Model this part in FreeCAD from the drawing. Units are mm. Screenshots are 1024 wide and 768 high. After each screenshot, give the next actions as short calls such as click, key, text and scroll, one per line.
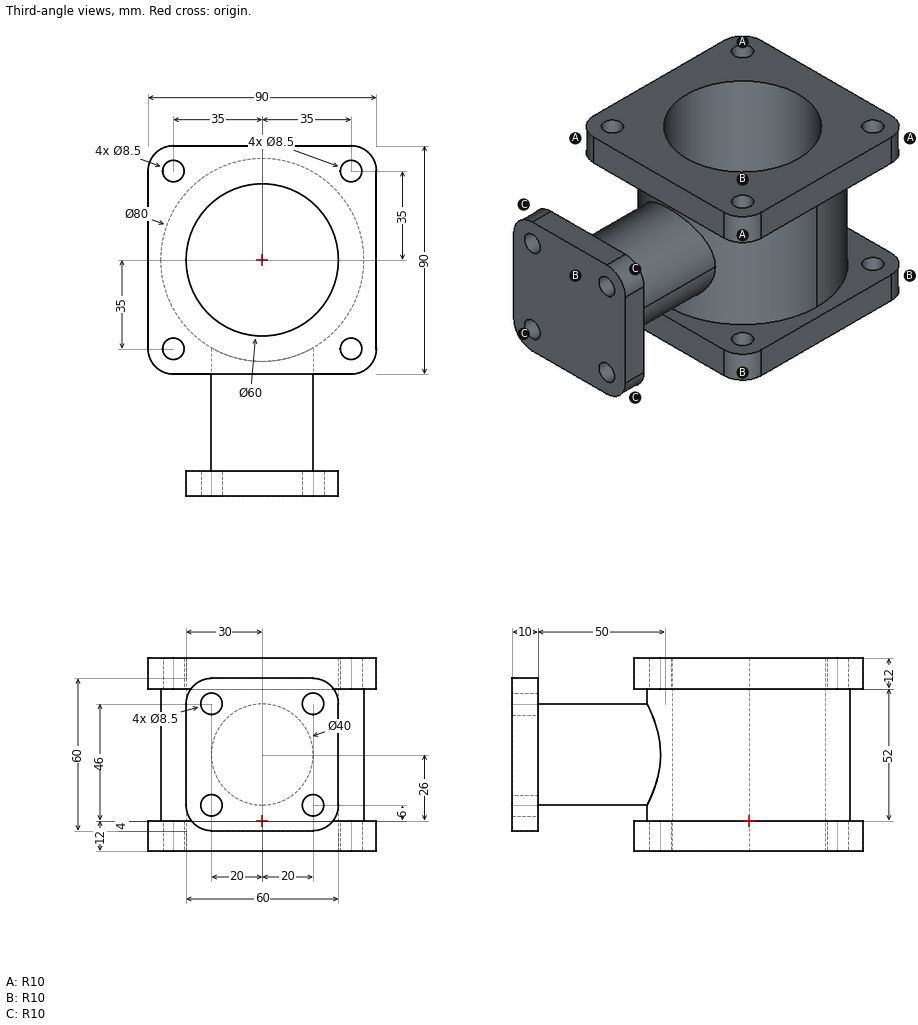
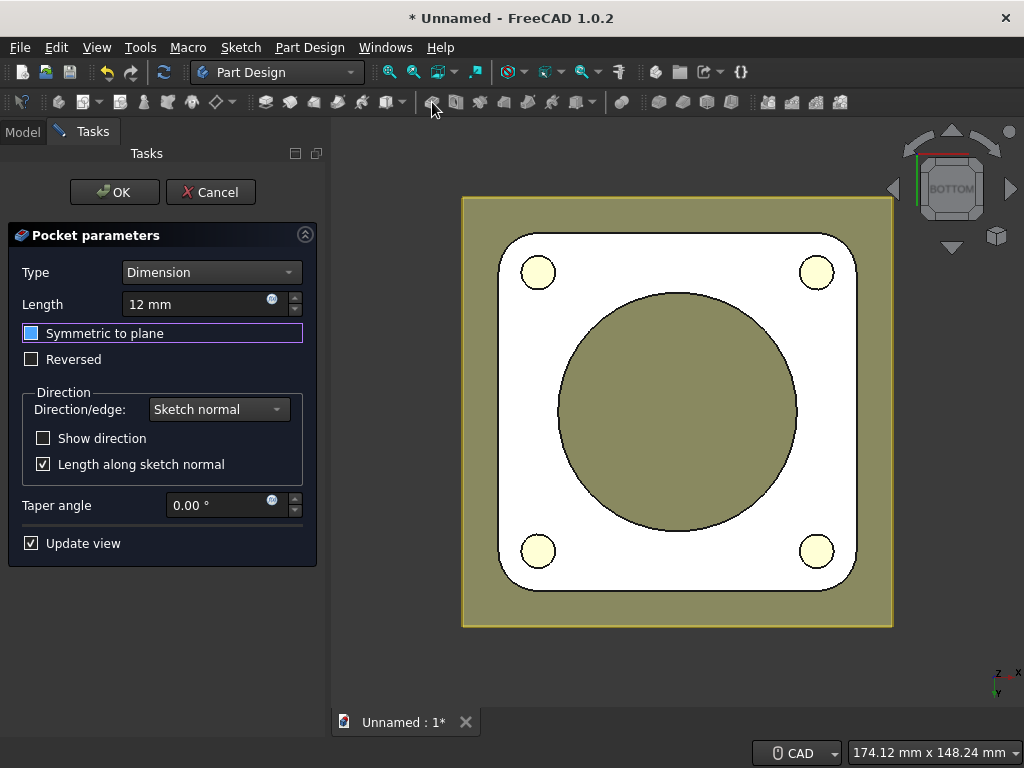
click(30, 359)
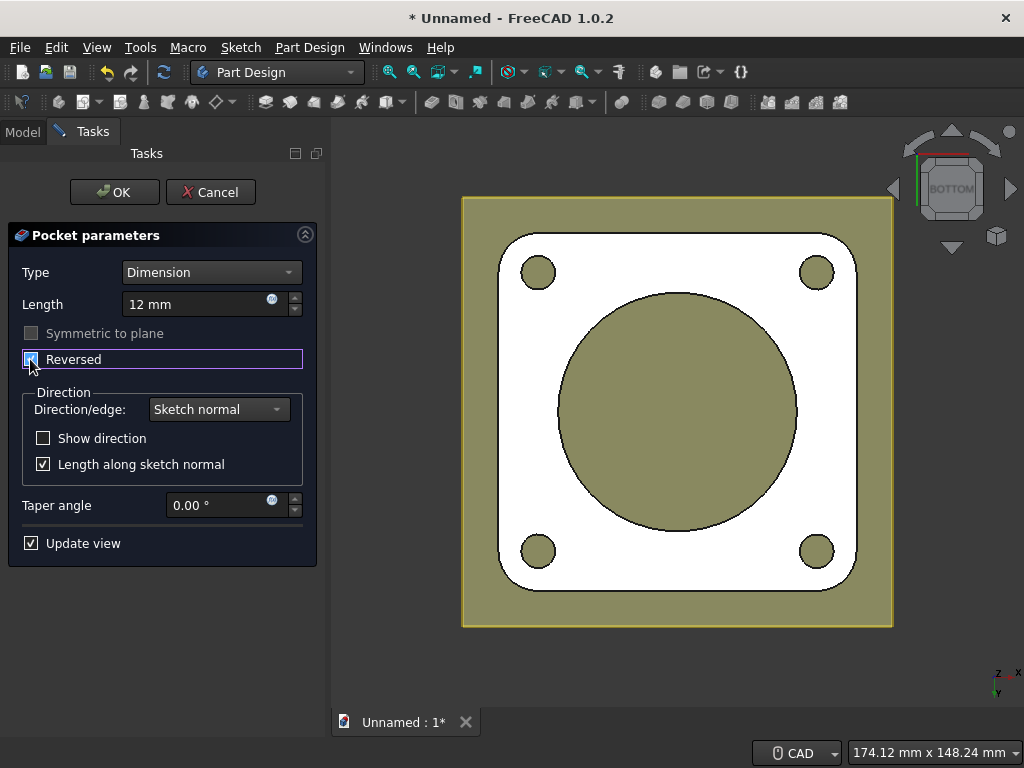
click(115, 192)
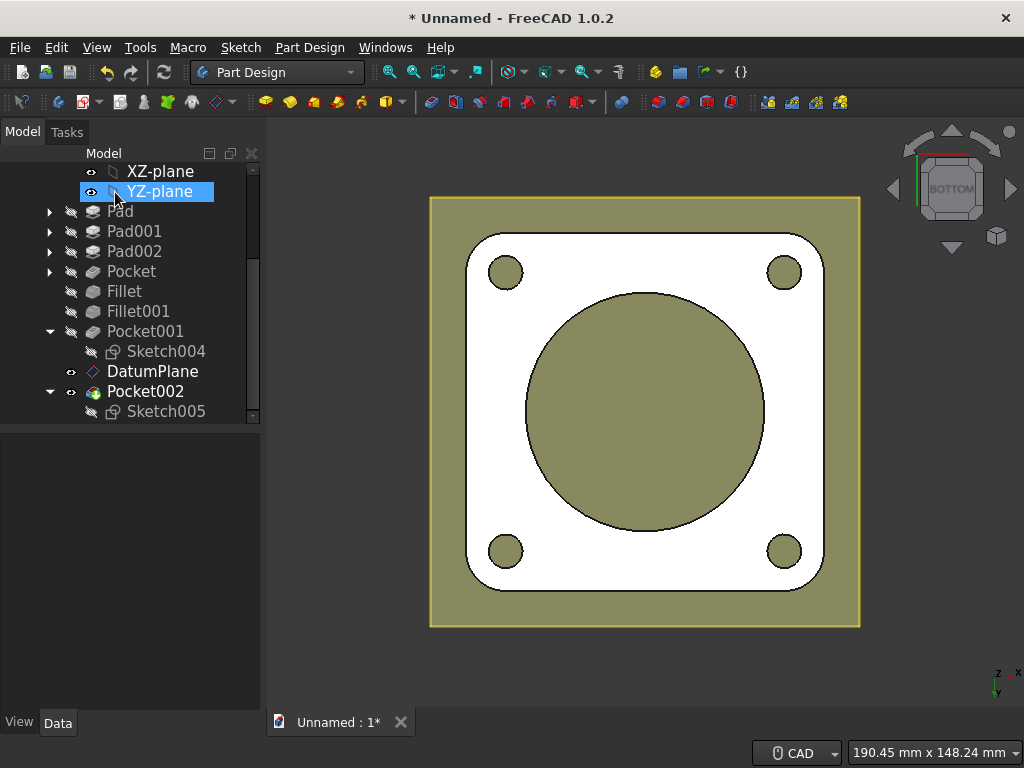
click(116, 372)
key(space)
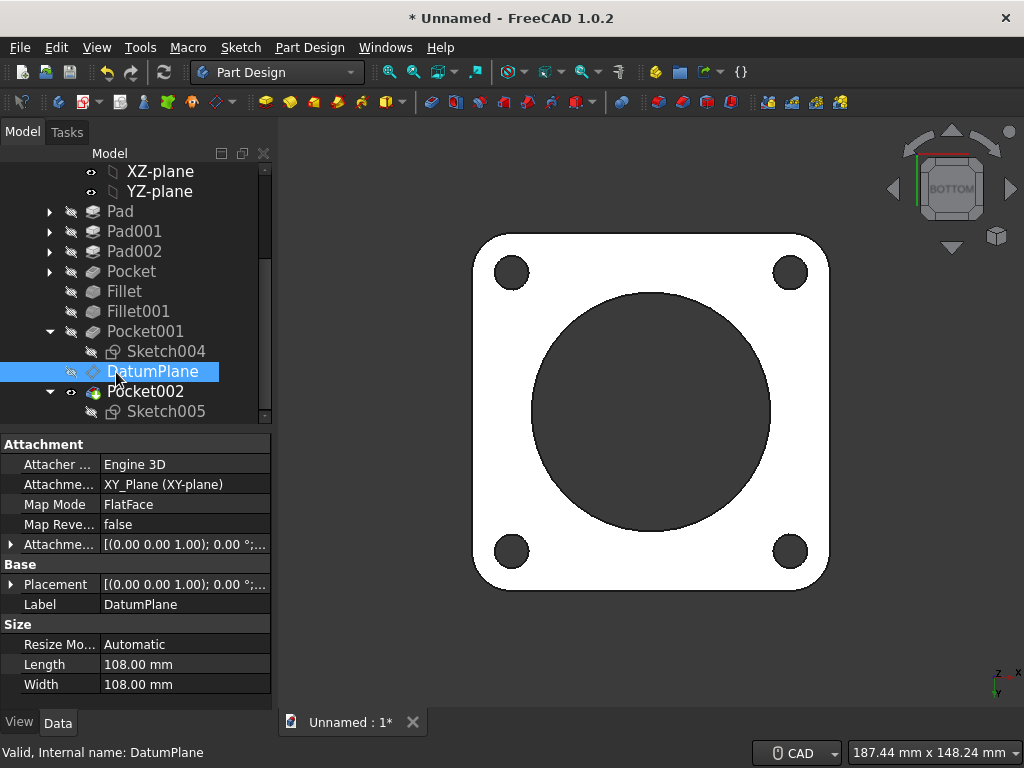
scroll(160, 287, down, 3)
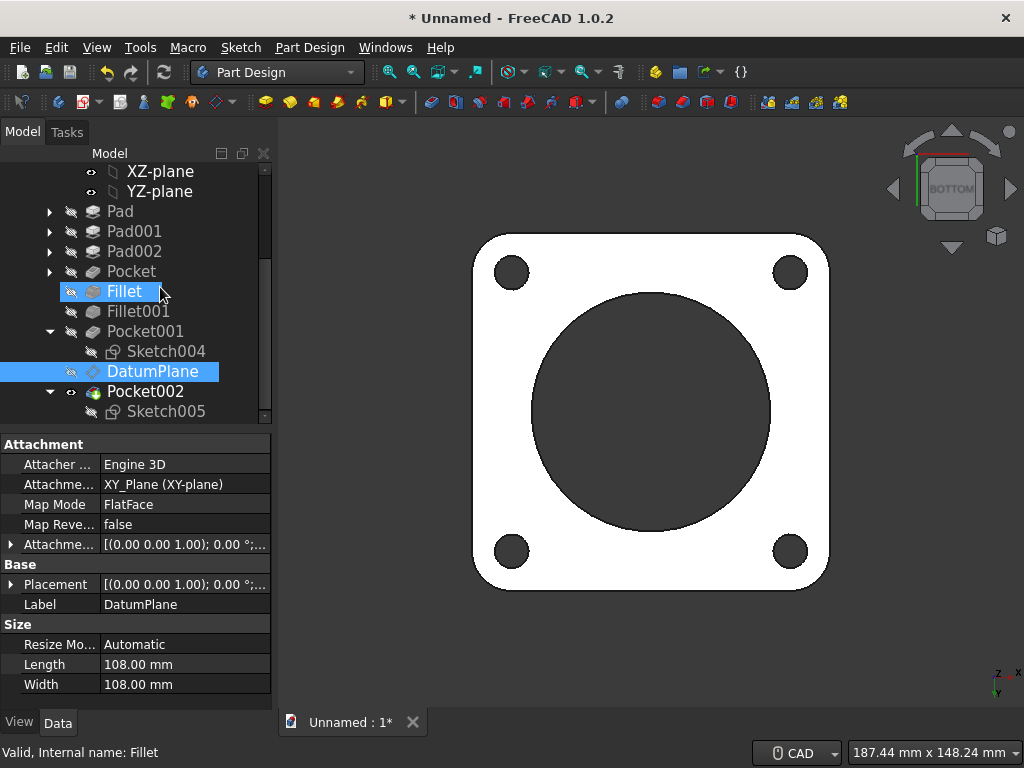
scroll(160, 287, up, 15)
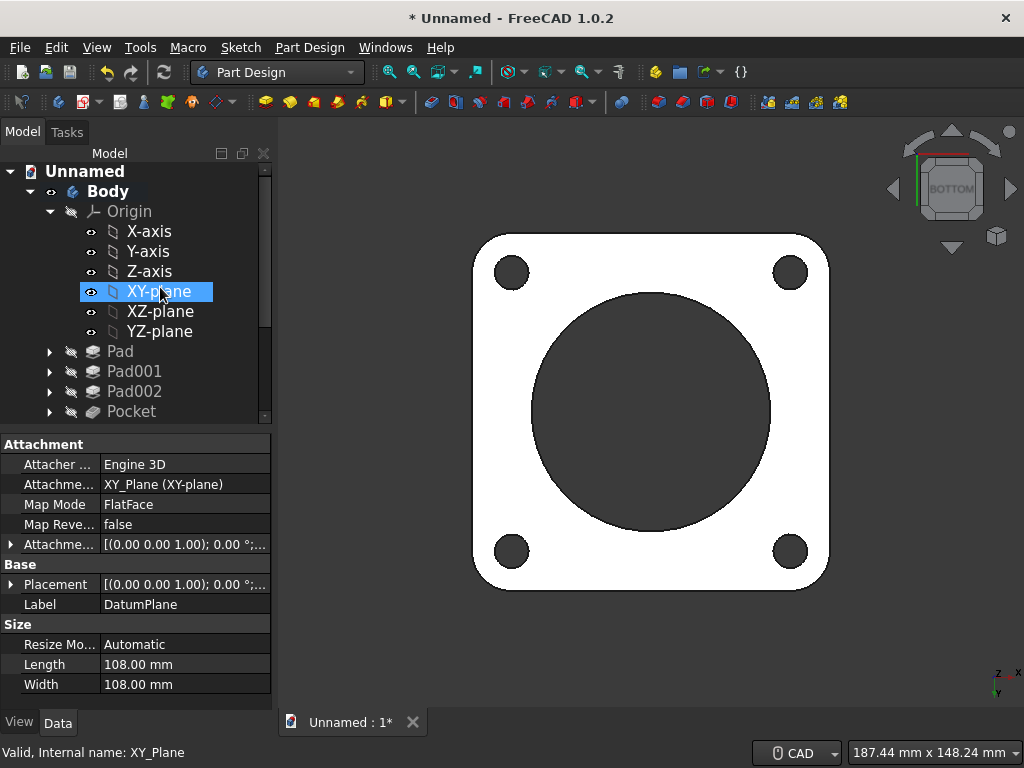
click(136, 312)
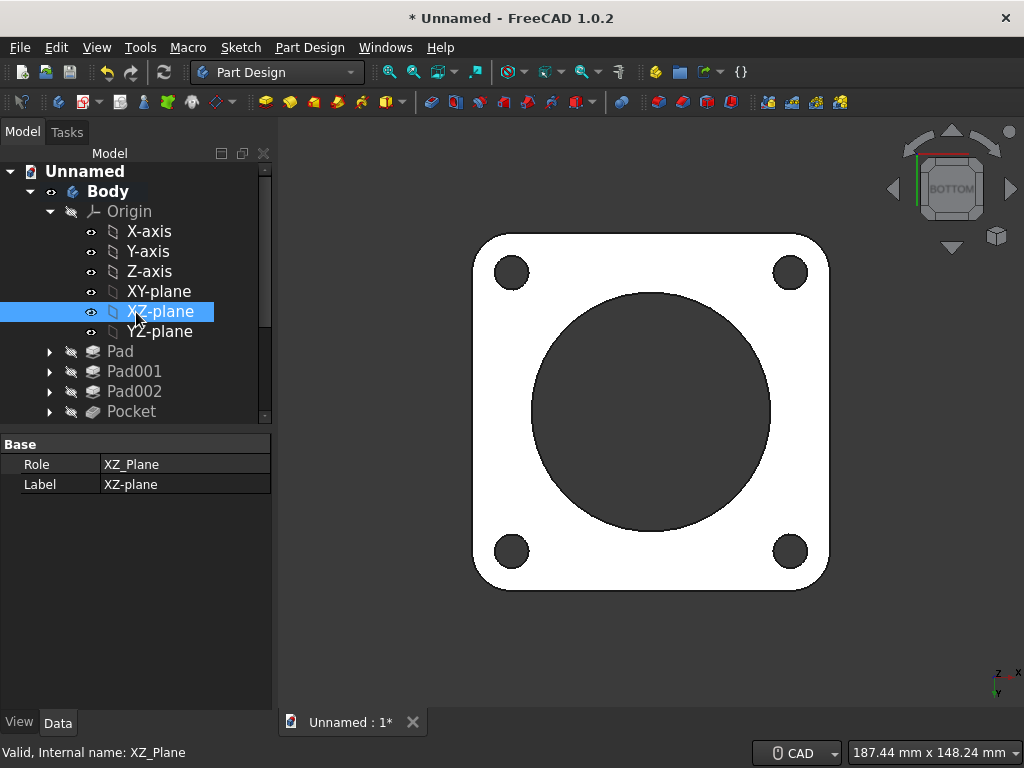
click(216, 102)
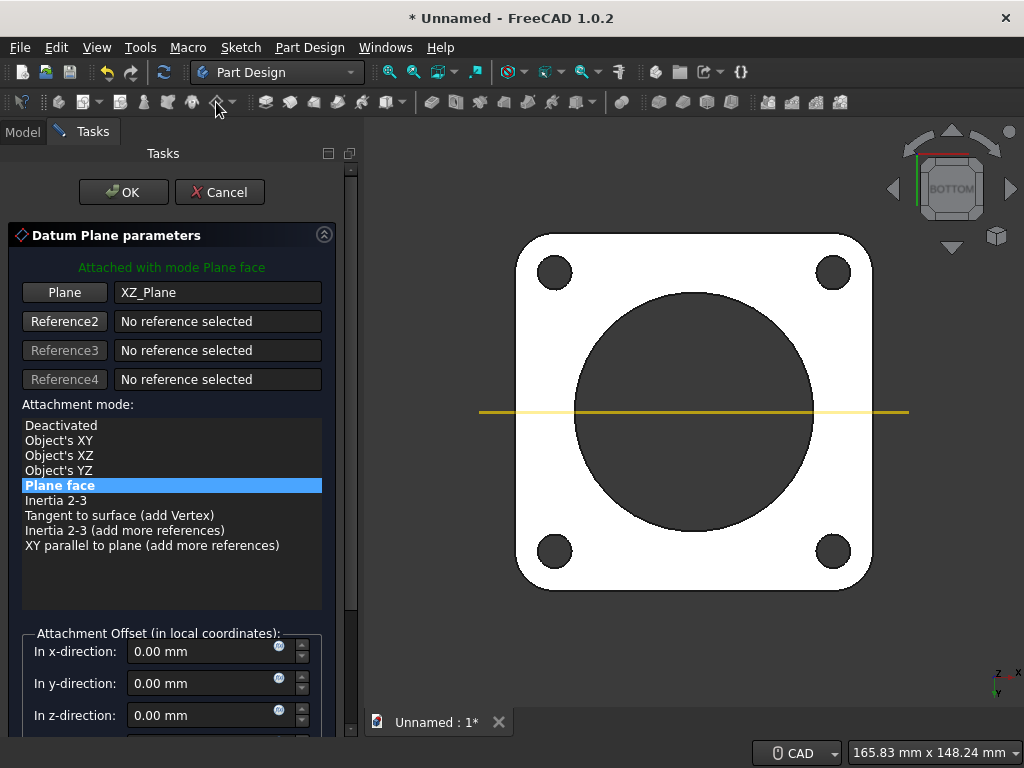
triple_click(210, 715)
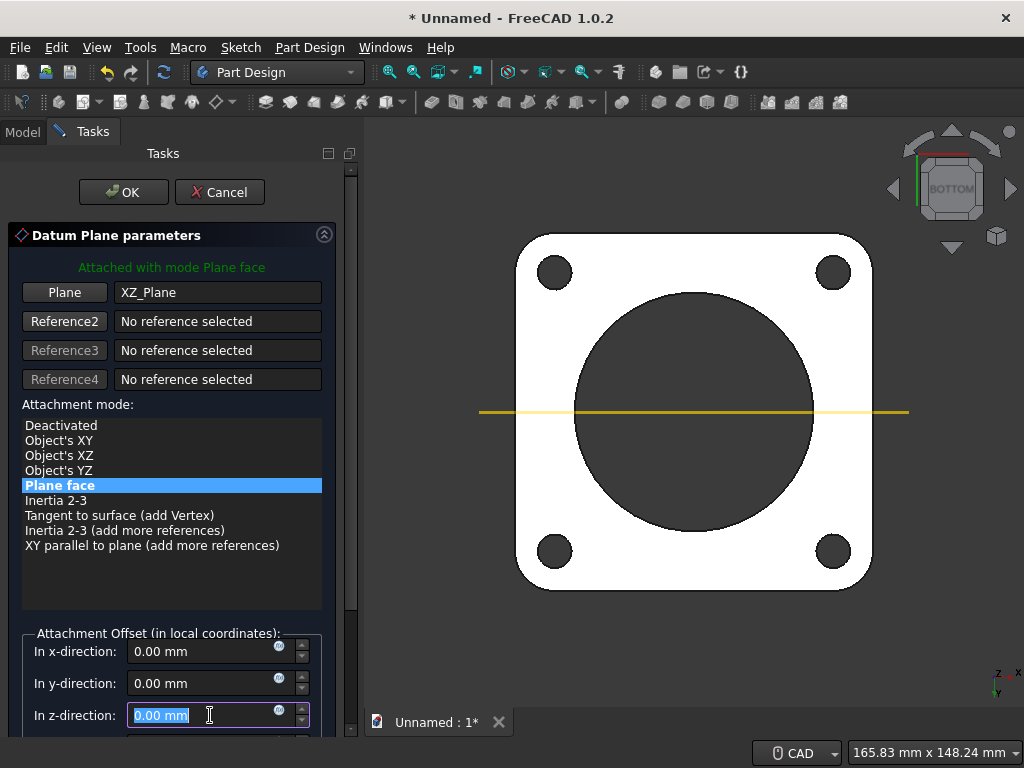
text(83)
key(Tab)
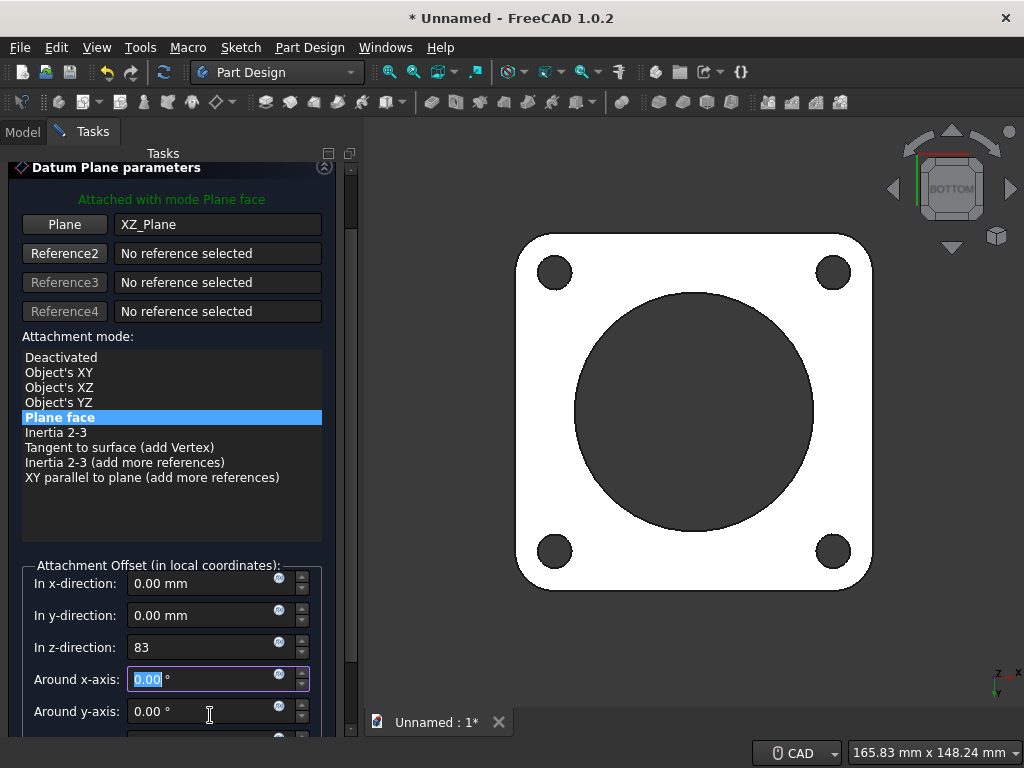
scroll(351, 450, up, 2)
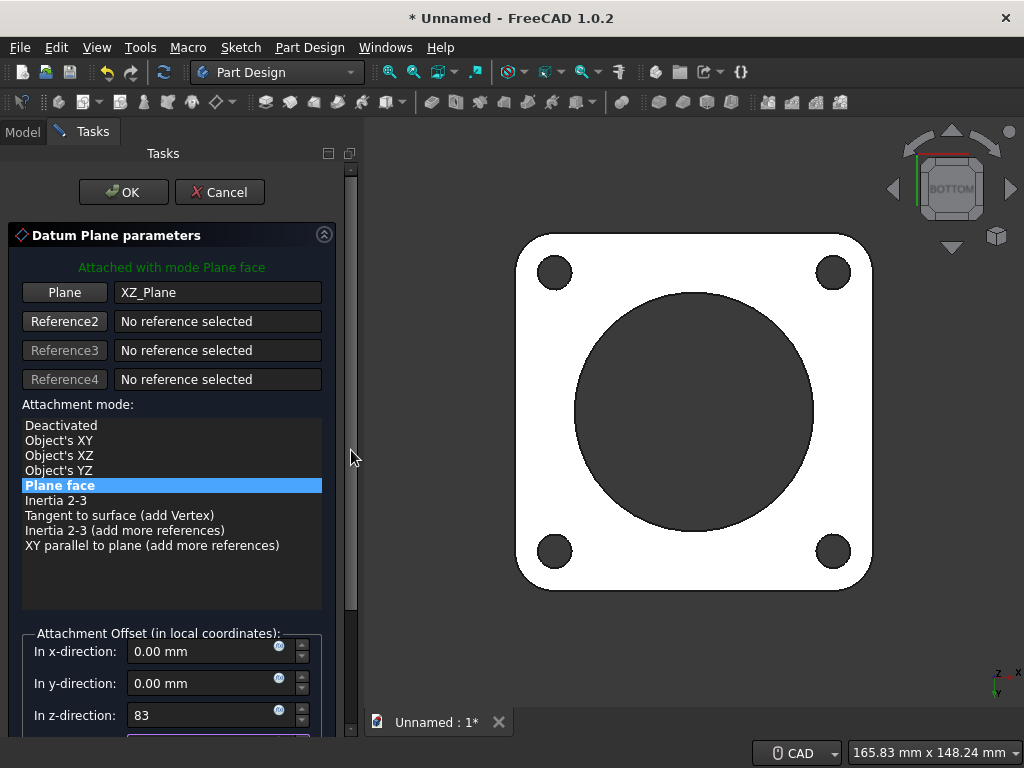
click(124, 192)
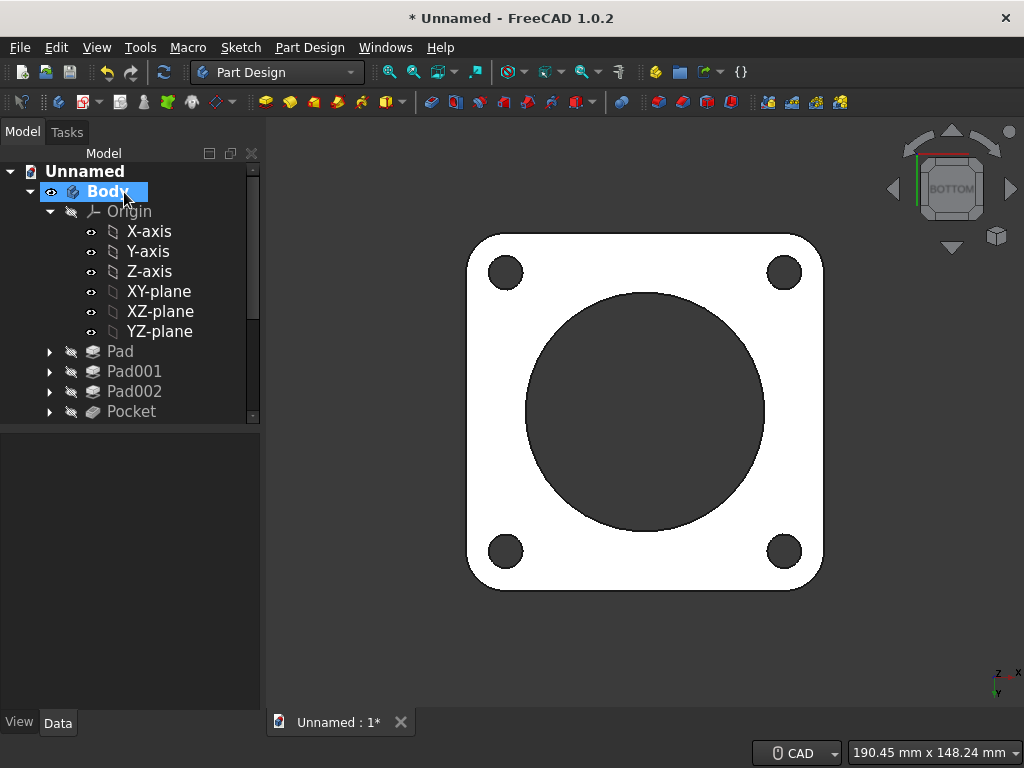
scroll(100, 287, down, 3)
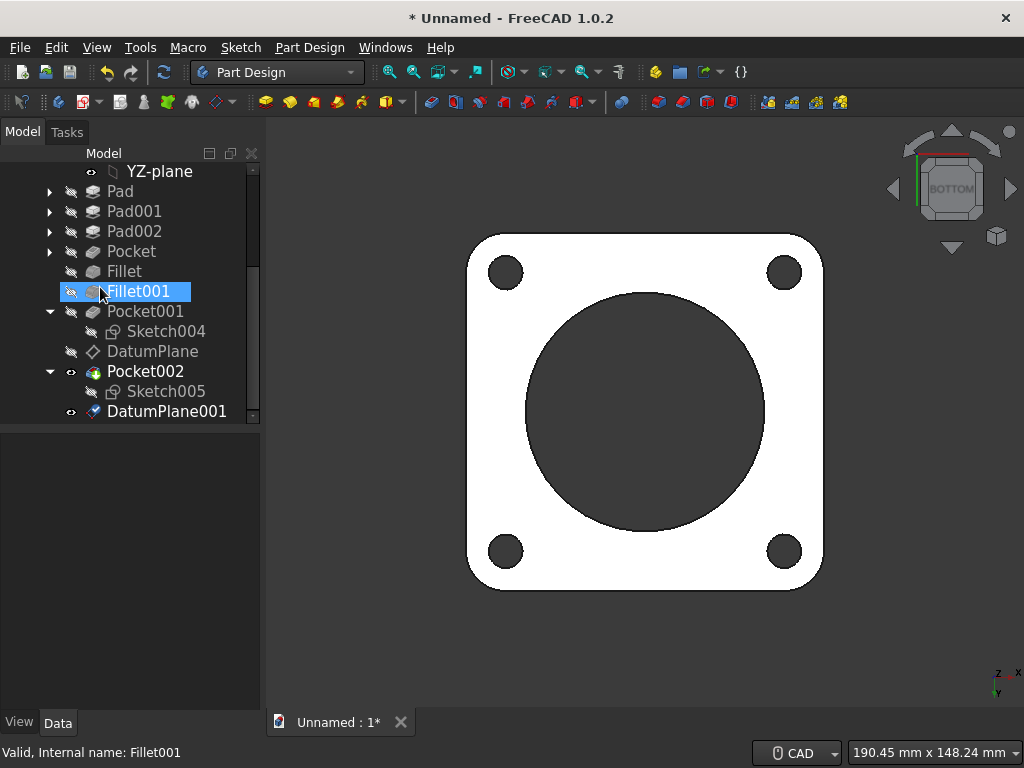
click(116, 412)